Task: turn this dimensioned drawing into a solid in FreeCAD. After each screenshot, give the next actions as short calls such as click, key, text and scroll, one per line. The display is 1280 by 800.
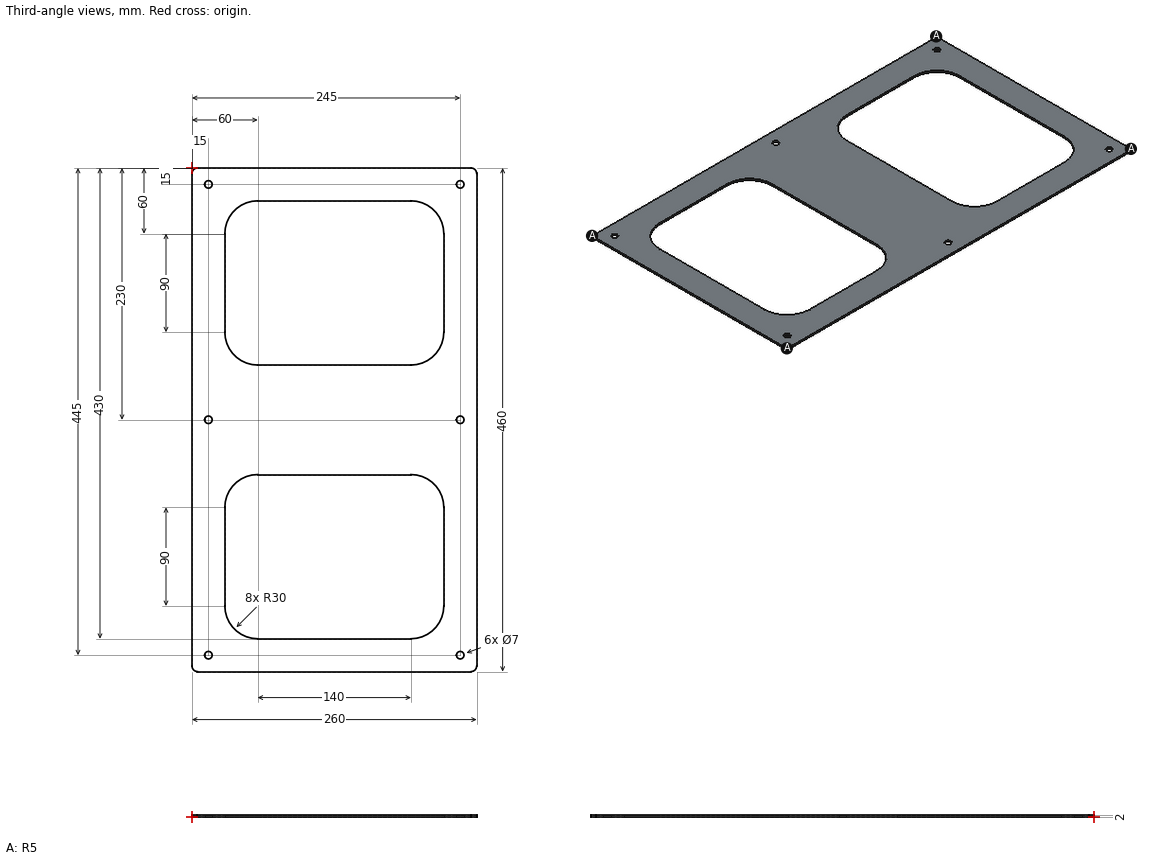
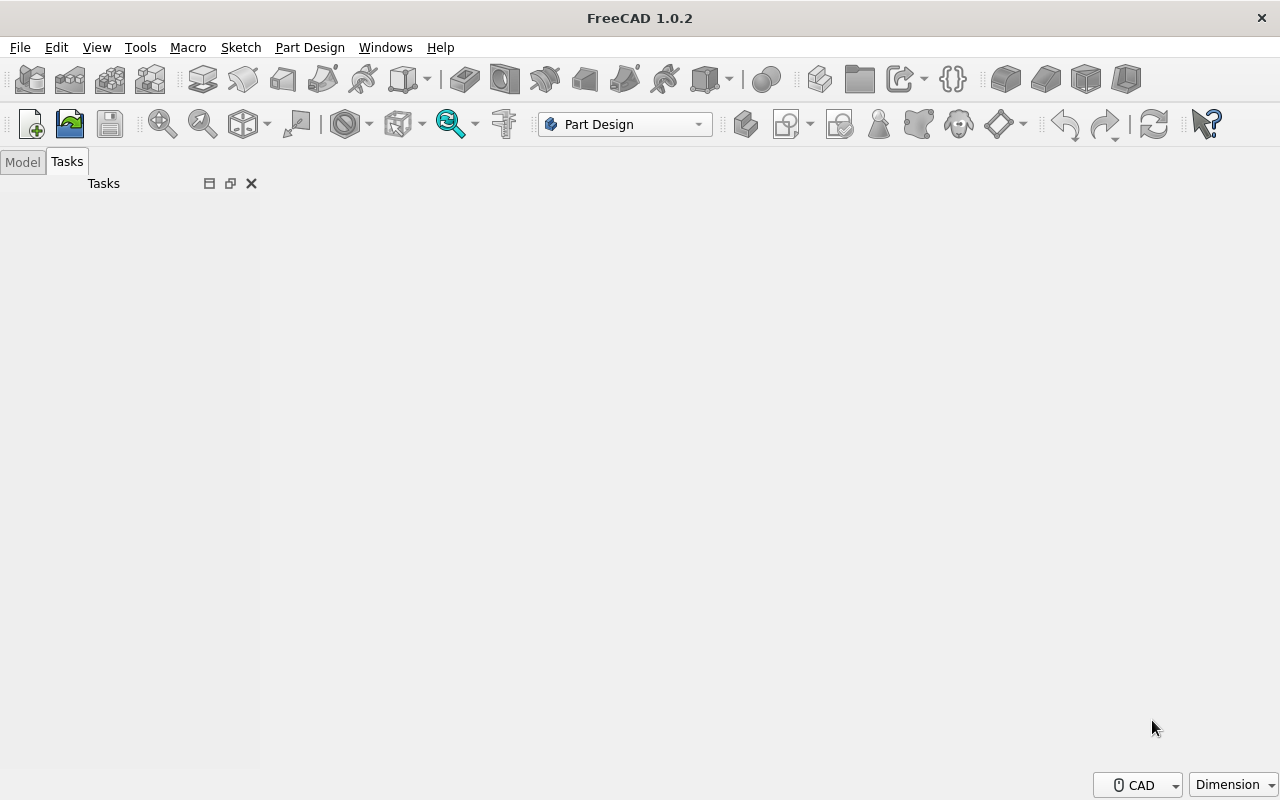
click(30, 124)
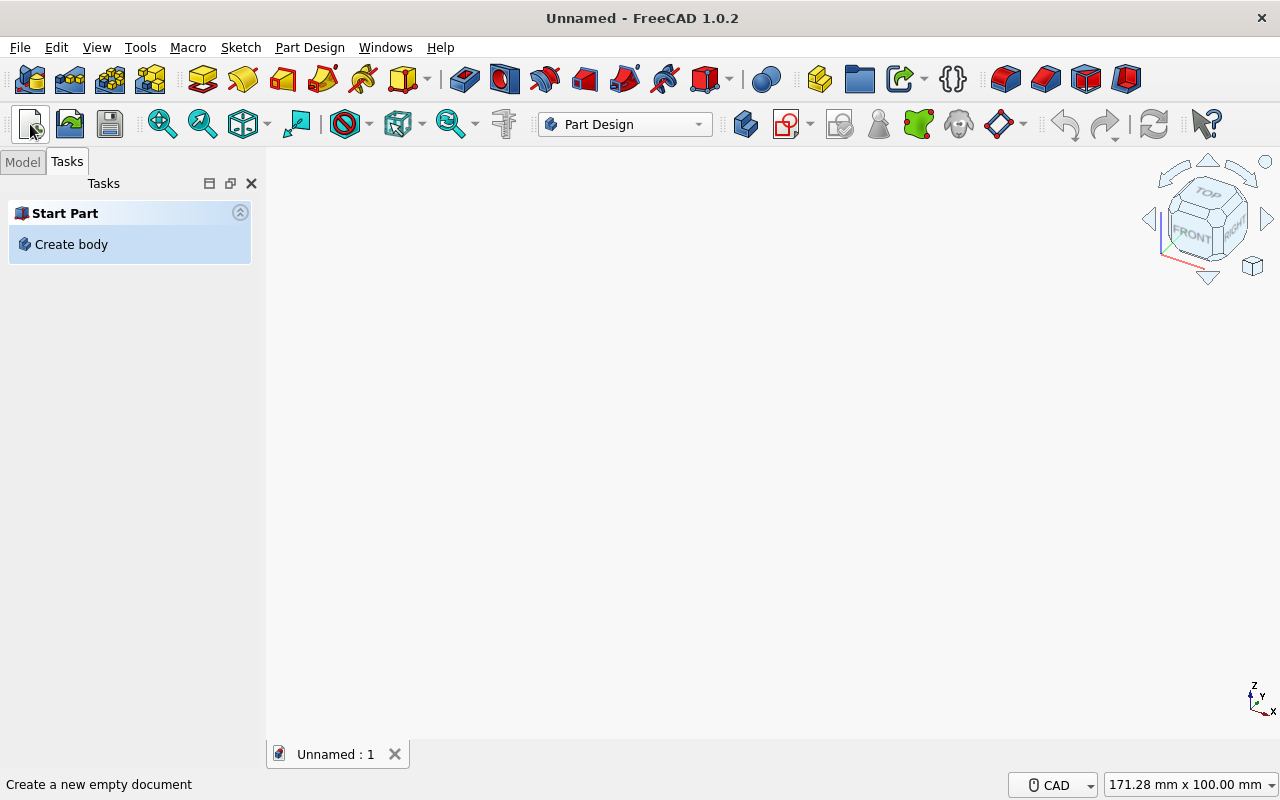
click(786, 124)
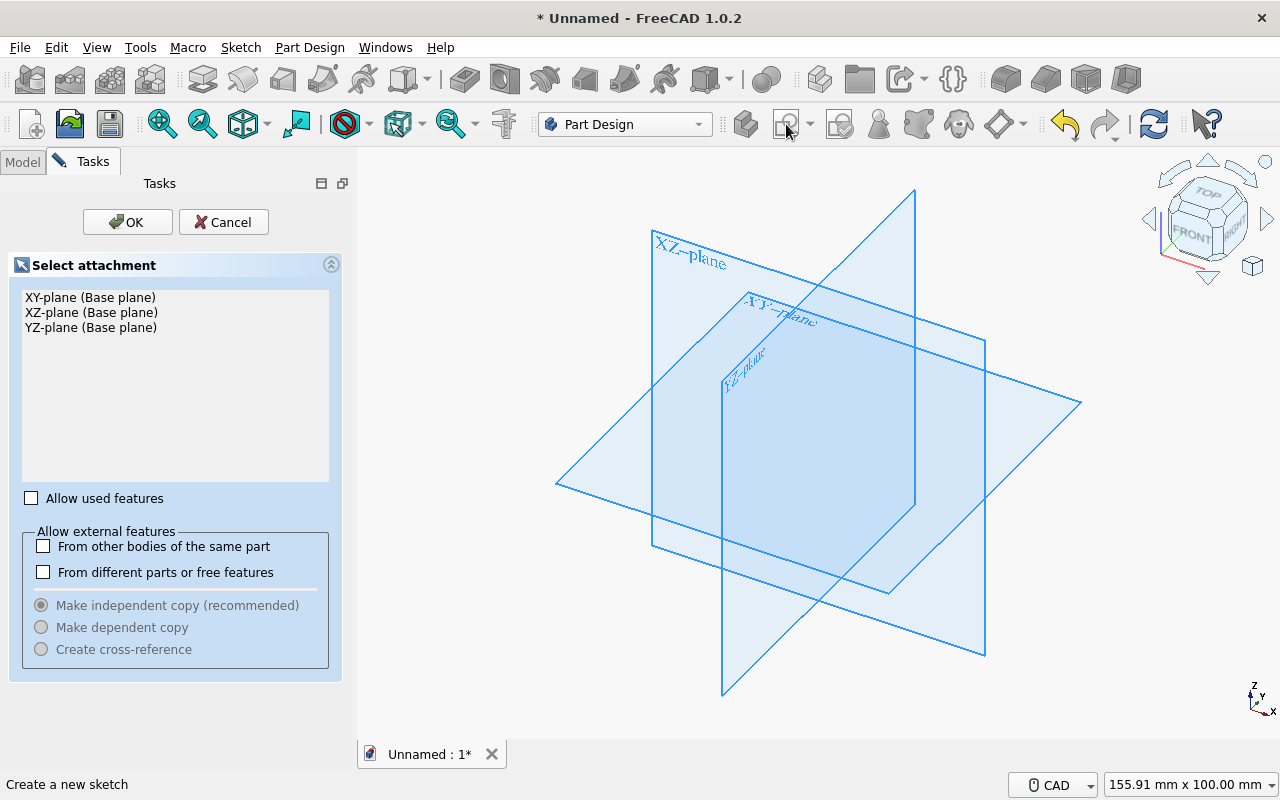
click(82, 298)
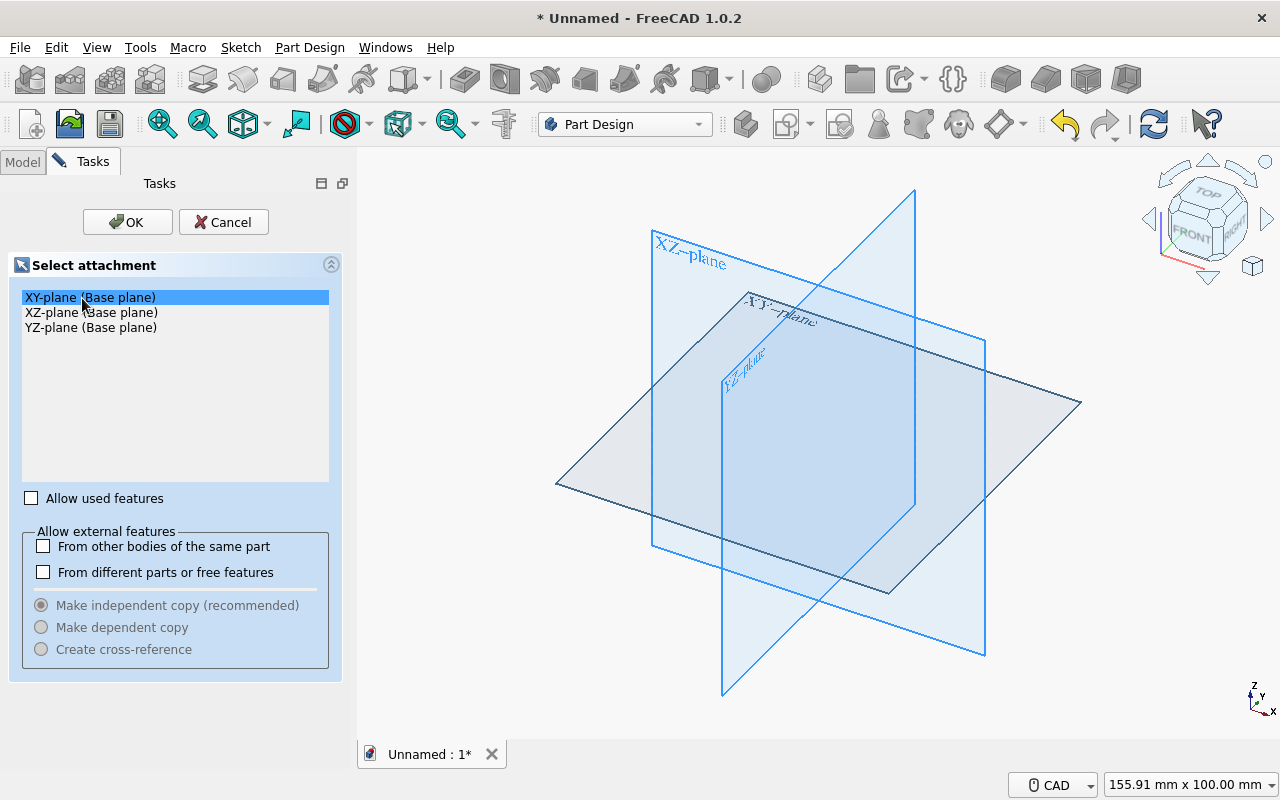
click(128, 222)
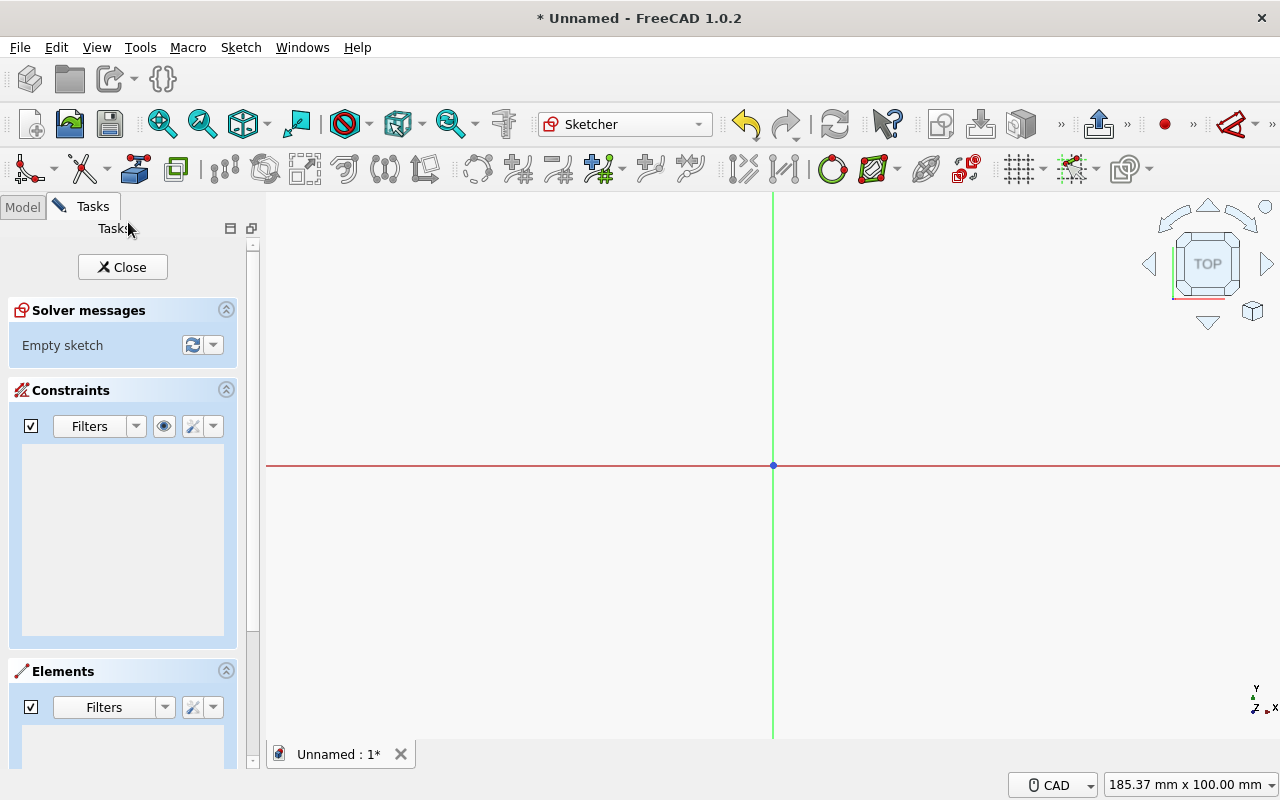
scroll(582, 269, down, 10)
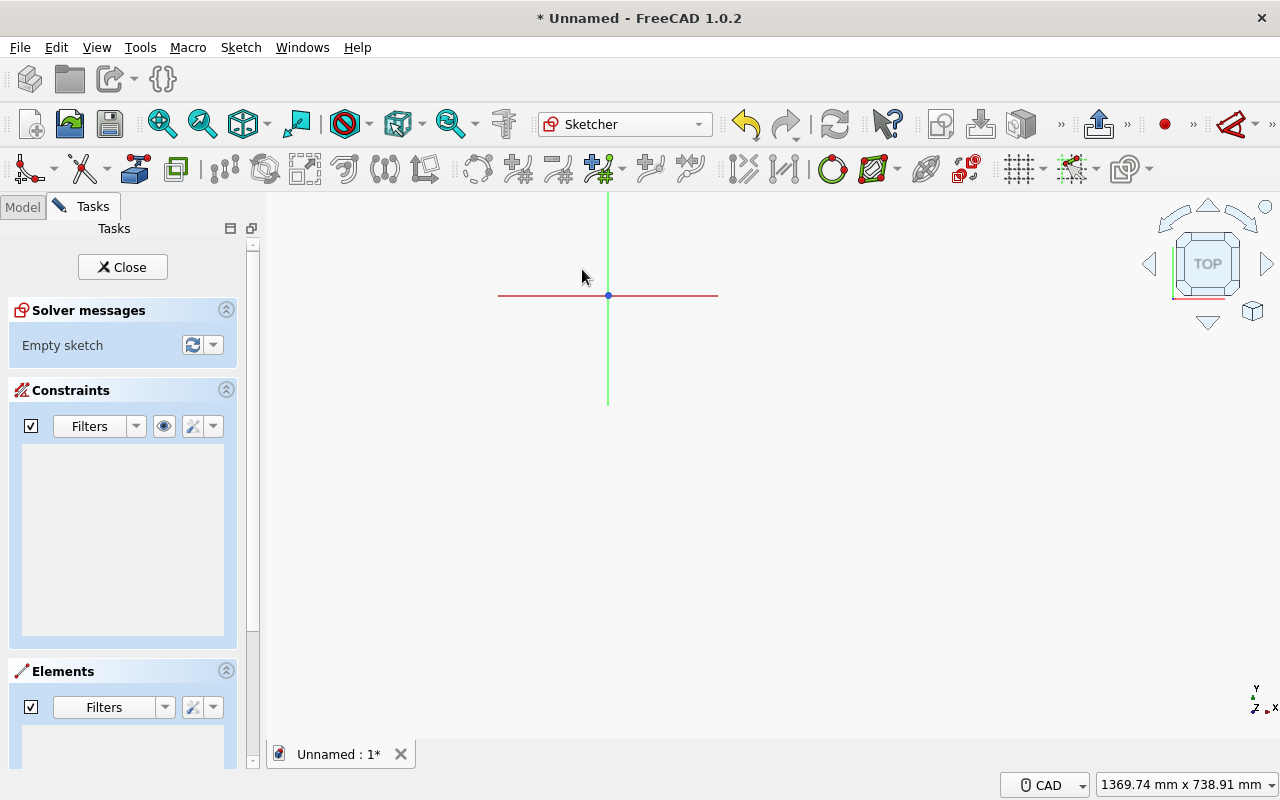
key(g)
key(r)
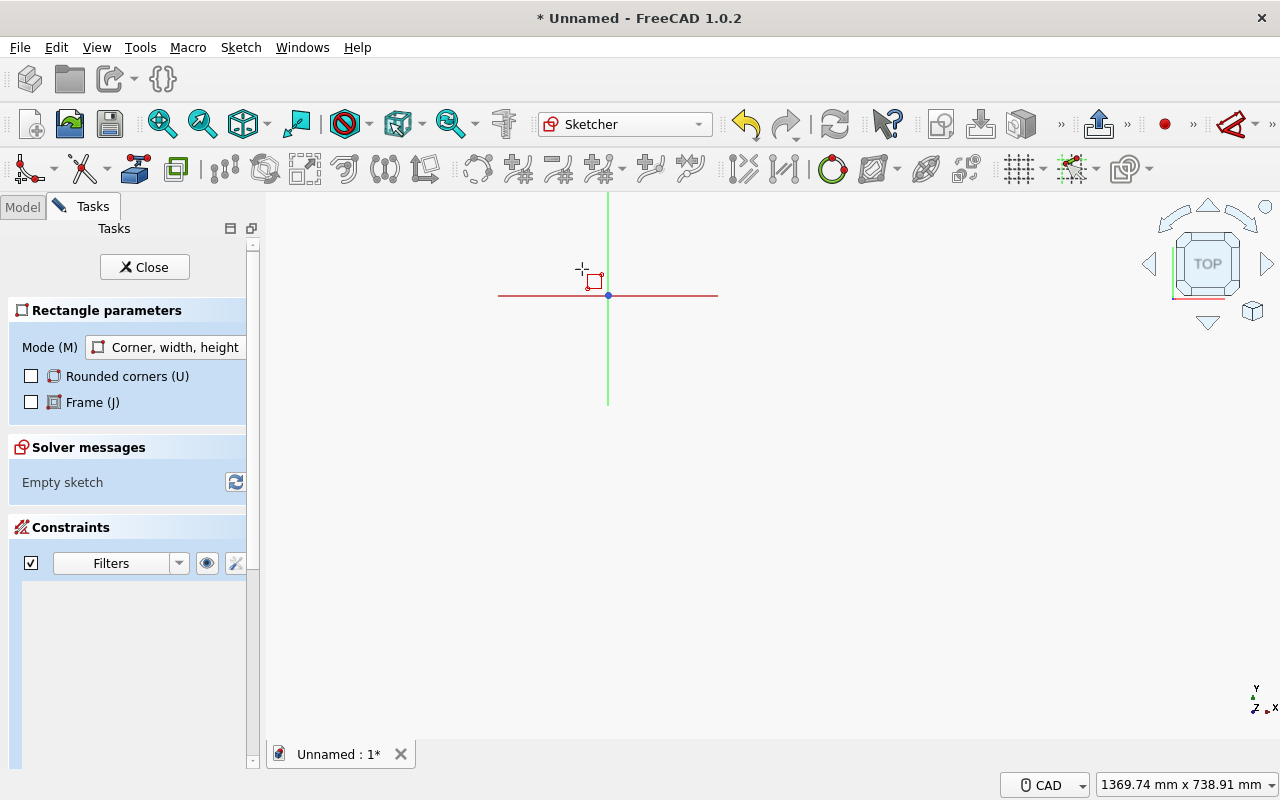
click(608, 296)
move(801, 636)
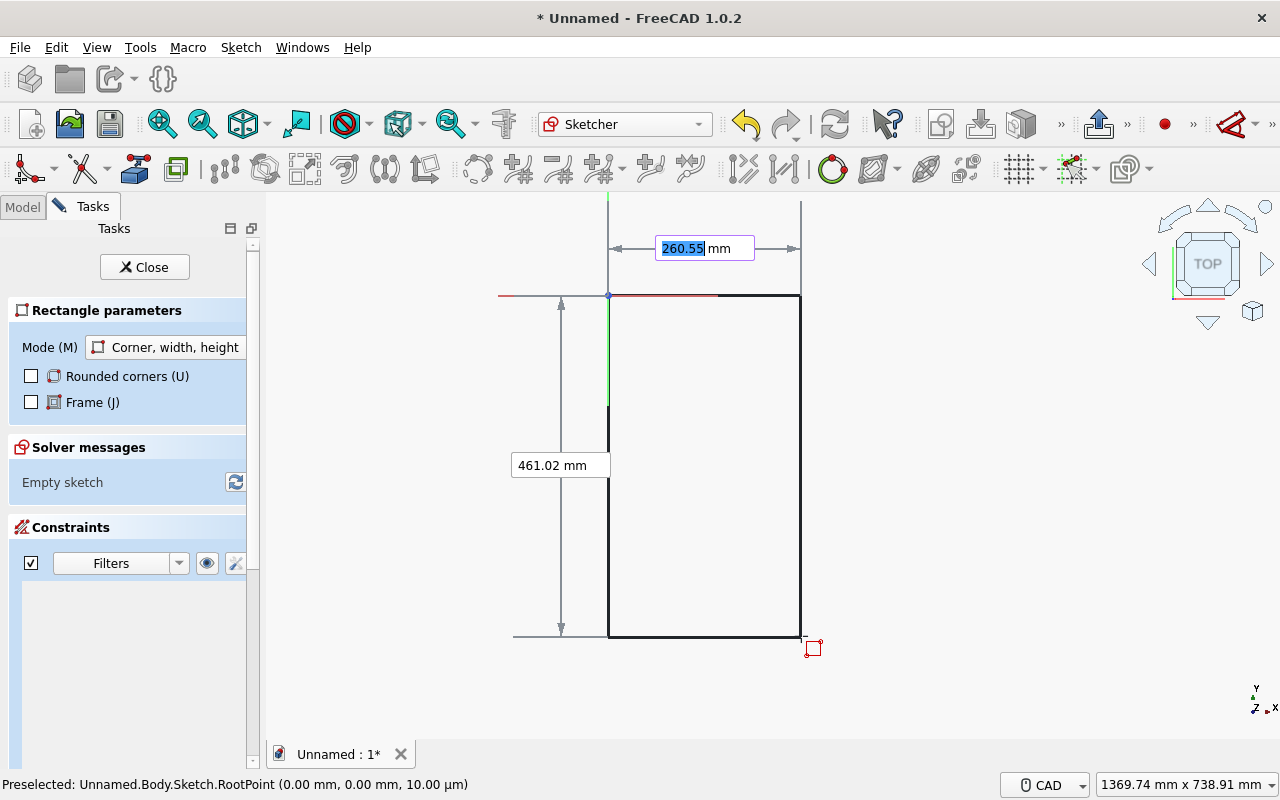
text(260)
key(Tab)
text(460)
key(Return)
key(Escape)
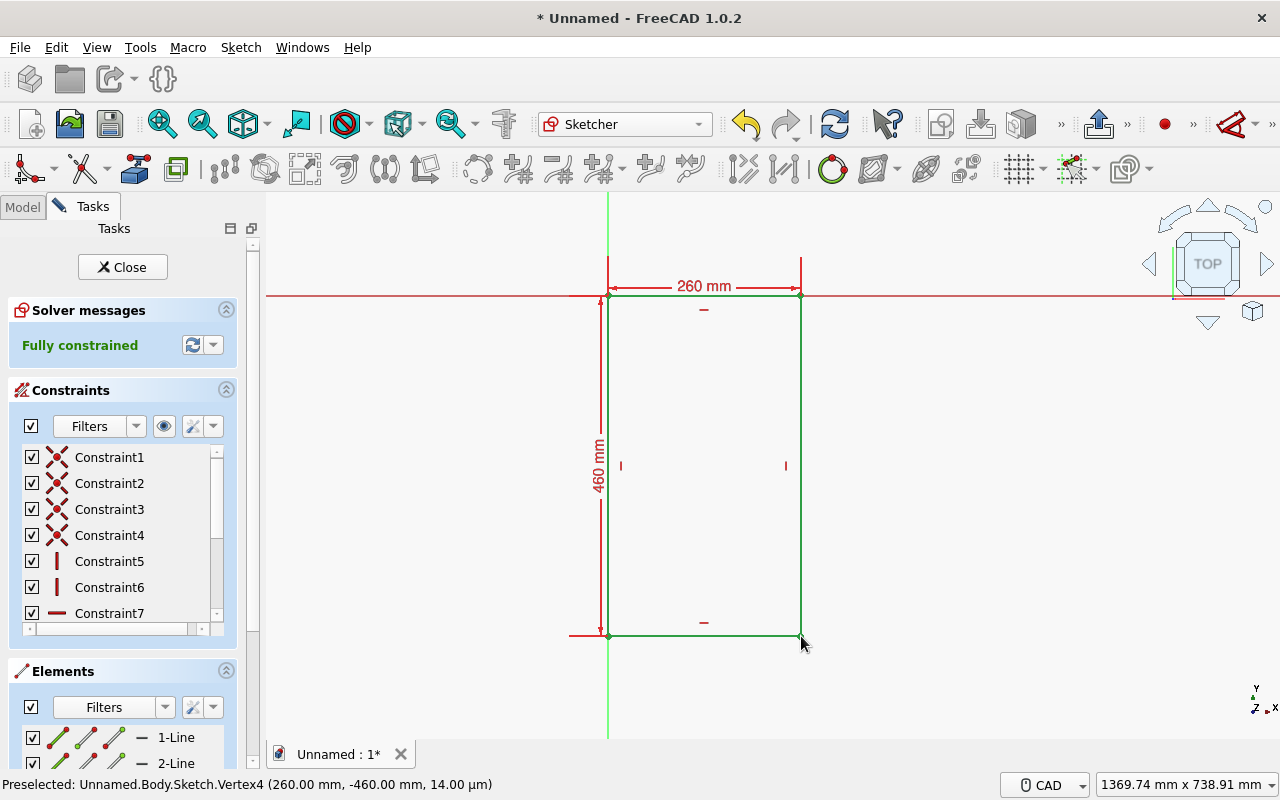
click(123, 267)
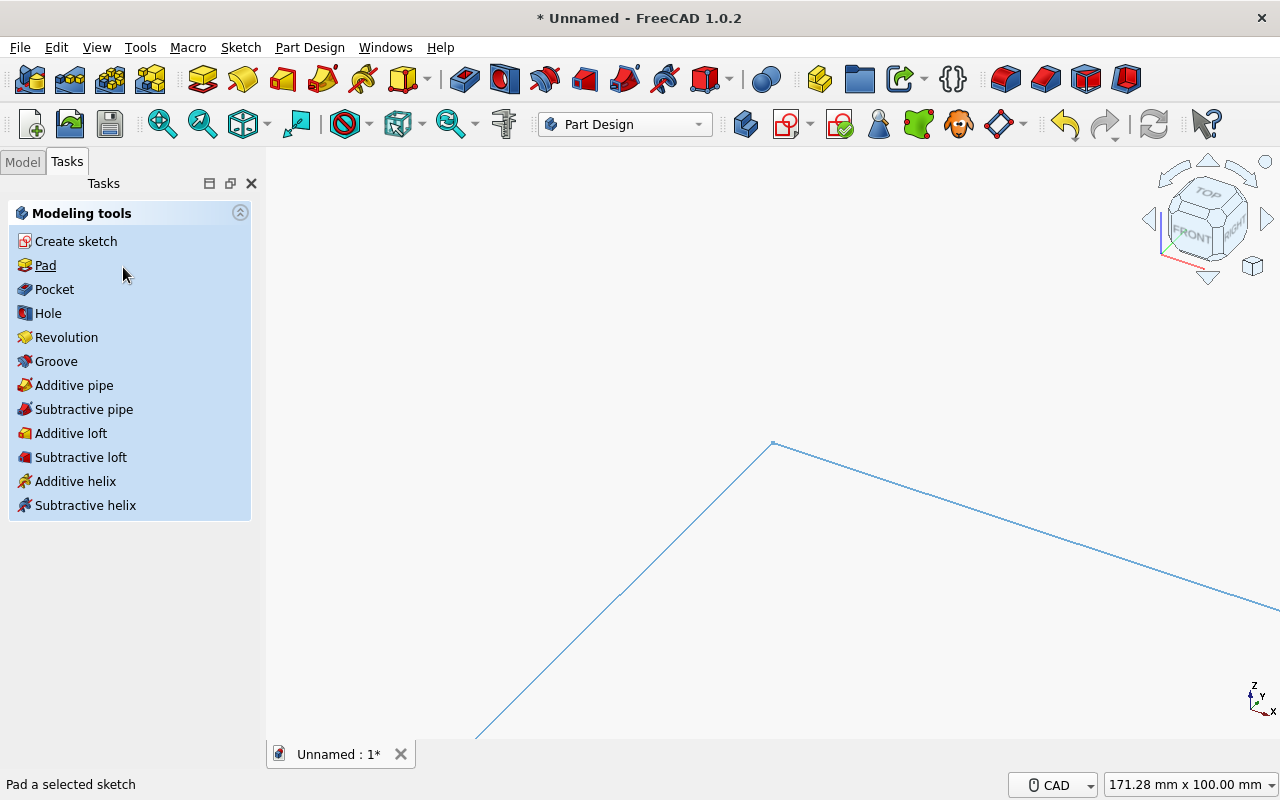
click(204, 80)